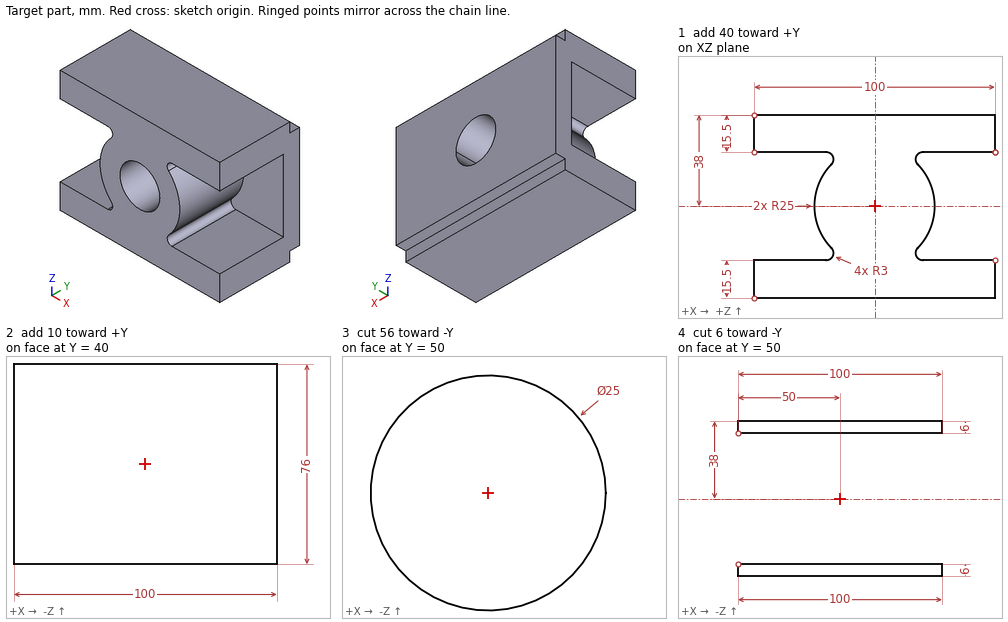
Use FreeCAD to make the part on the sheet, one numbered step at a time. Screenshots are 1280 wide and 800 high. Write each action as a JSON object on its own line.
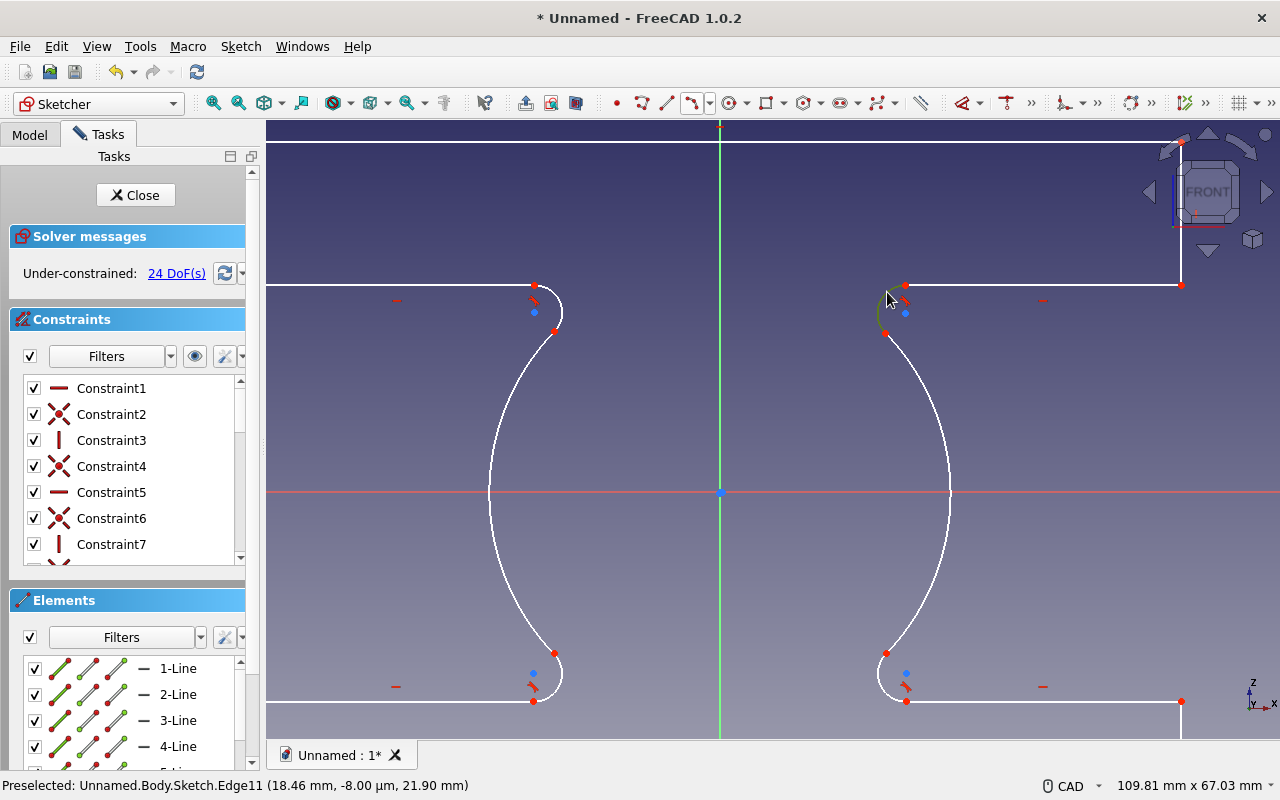
{"action": "left_click", "coordinate": [940, 563]}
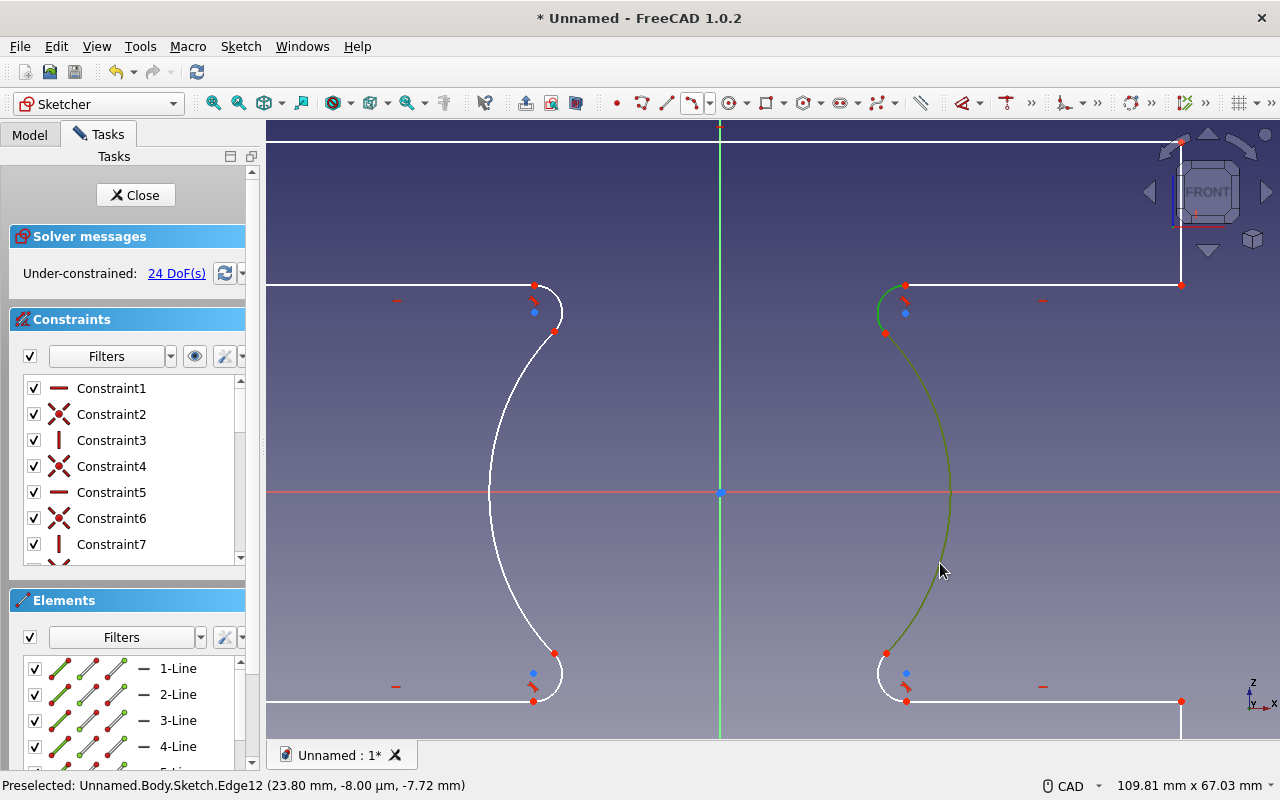
{"action": "key", "text": "t"}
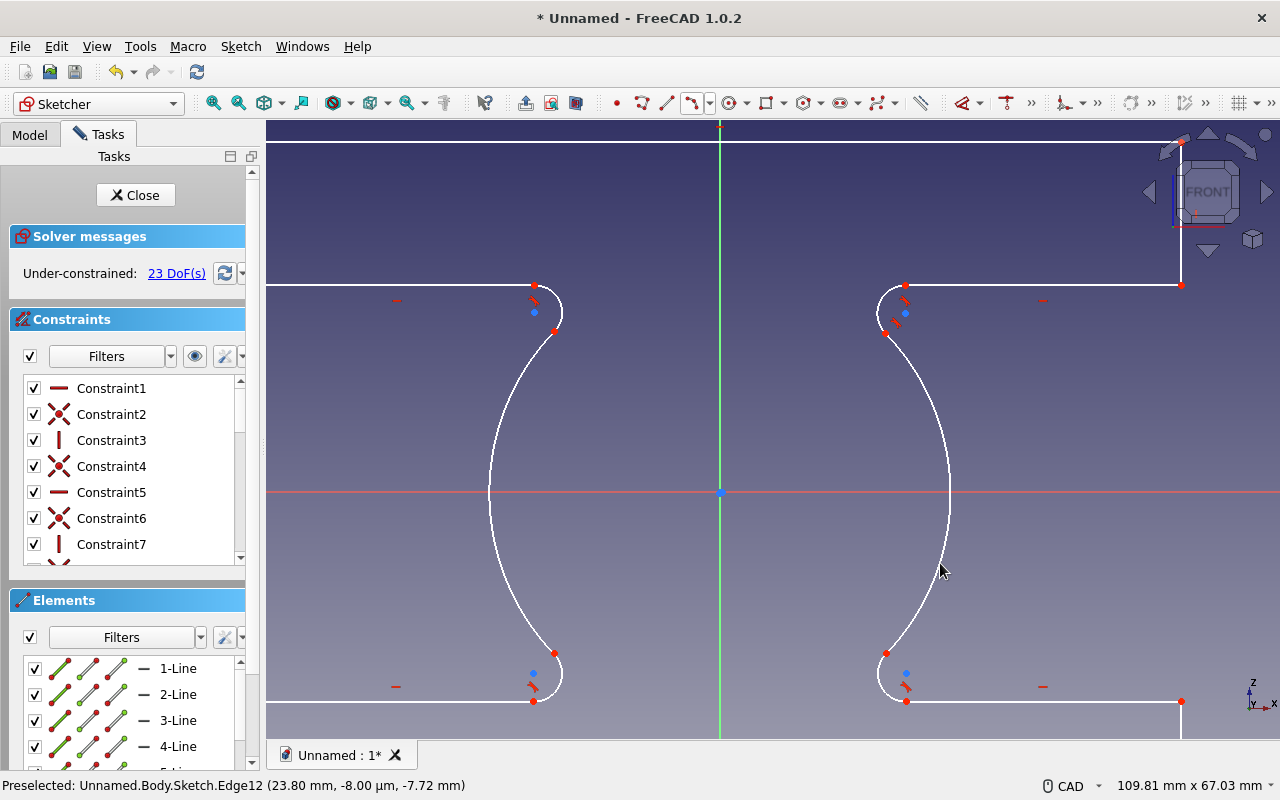
{"action": "left_click", "coordinate": [940, 563]}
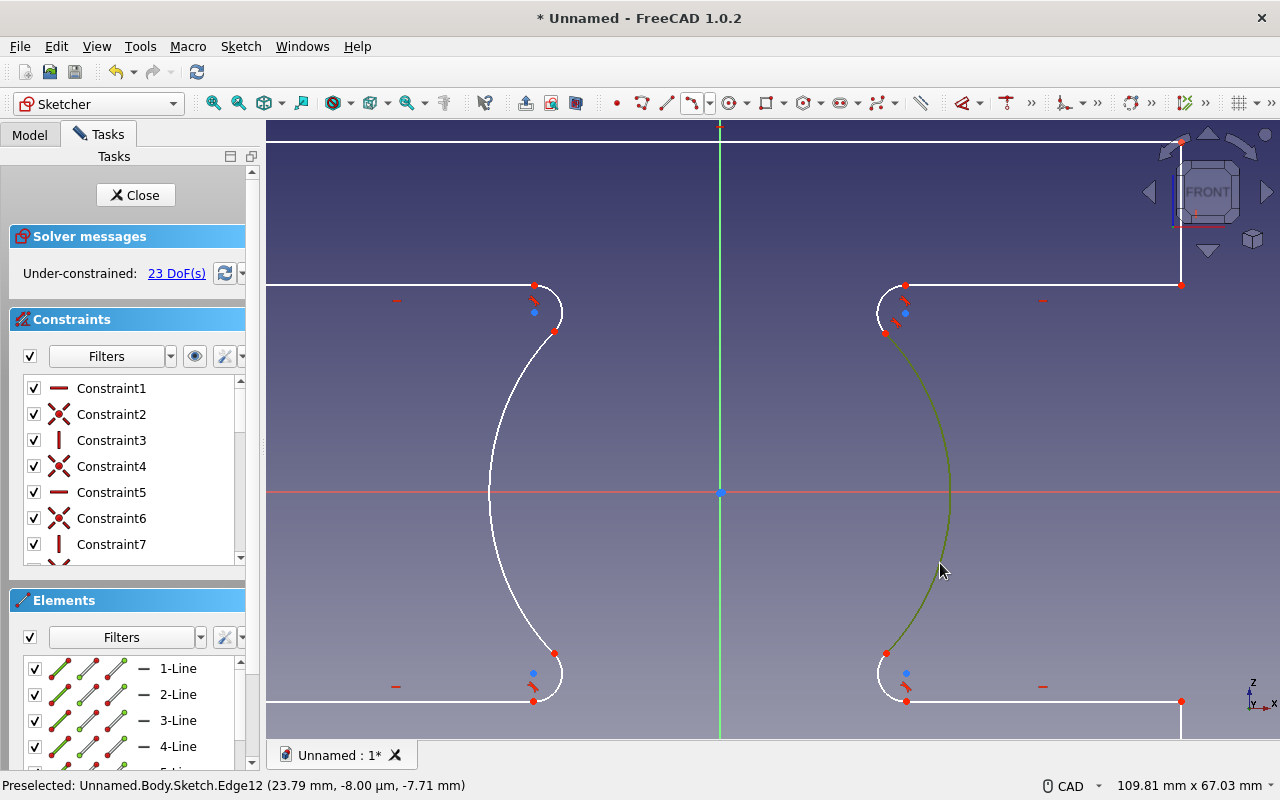
{"action": "left_click", "coordinate": [878, 672]}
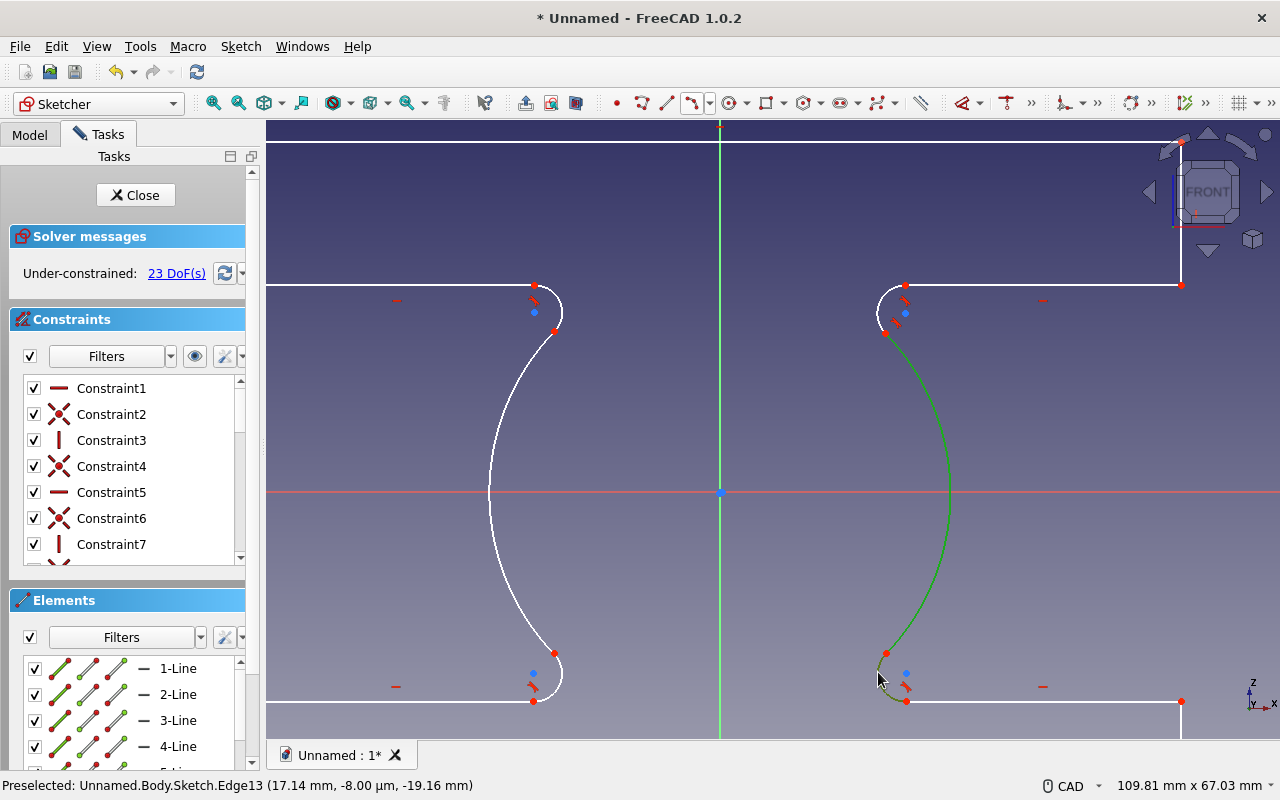
{"action": "key", "text": "t"}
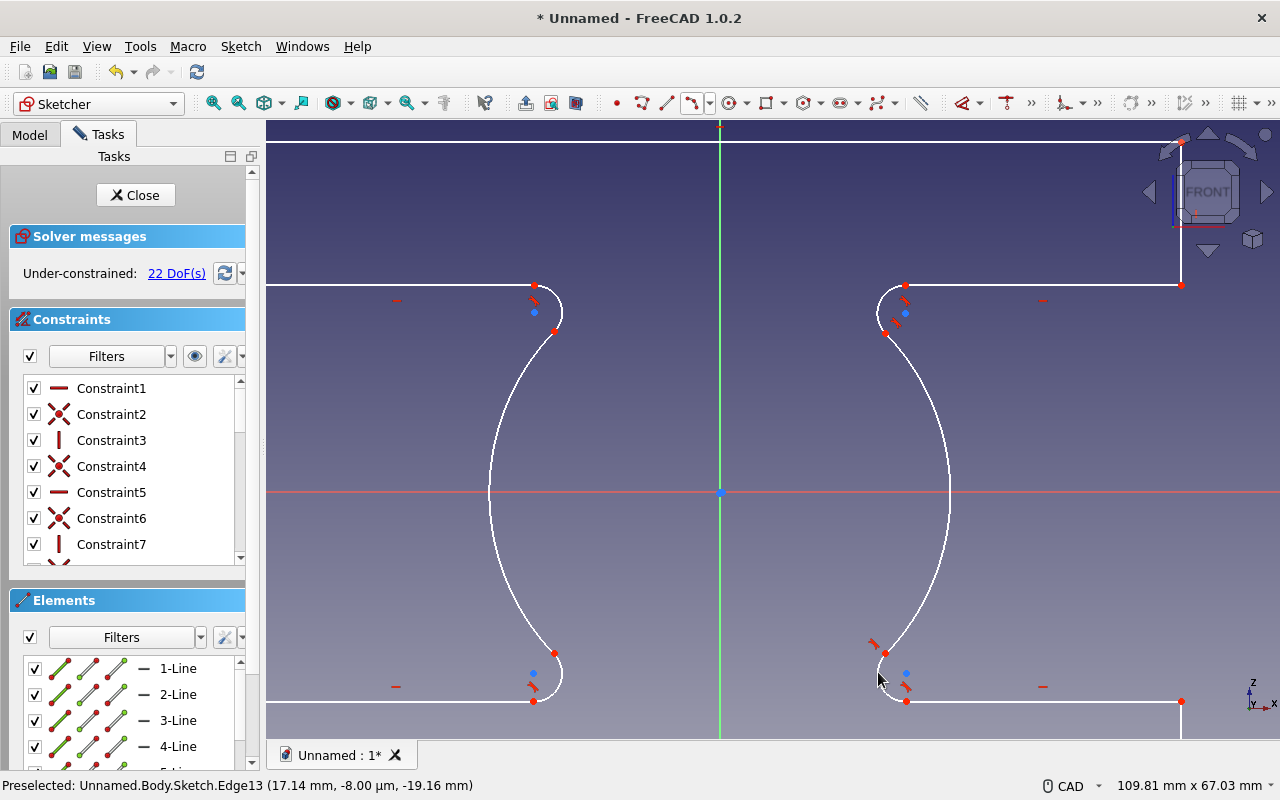
{"action": "left_click", "coordinate": [552, 695]}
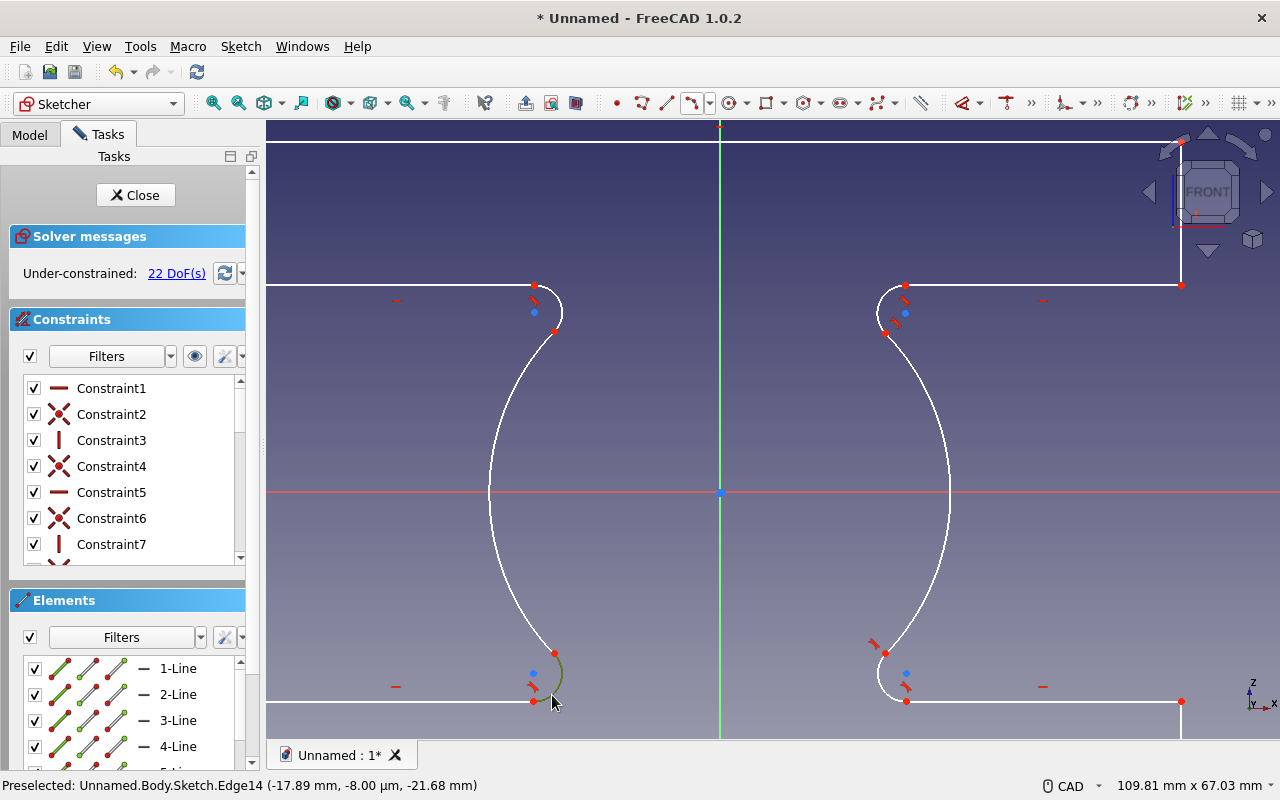
{"action": "left_click", "coordinate": [500, 423]}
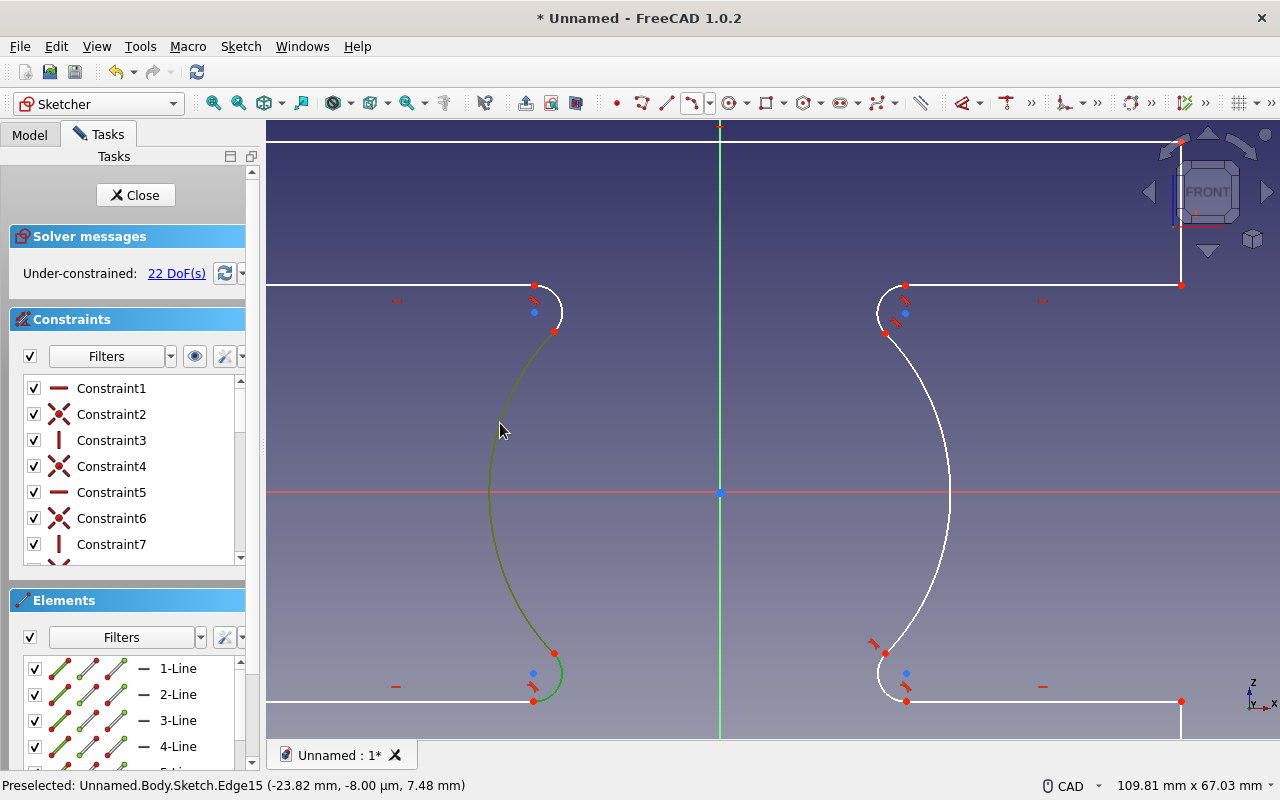
{"action": "key", "text": "t"}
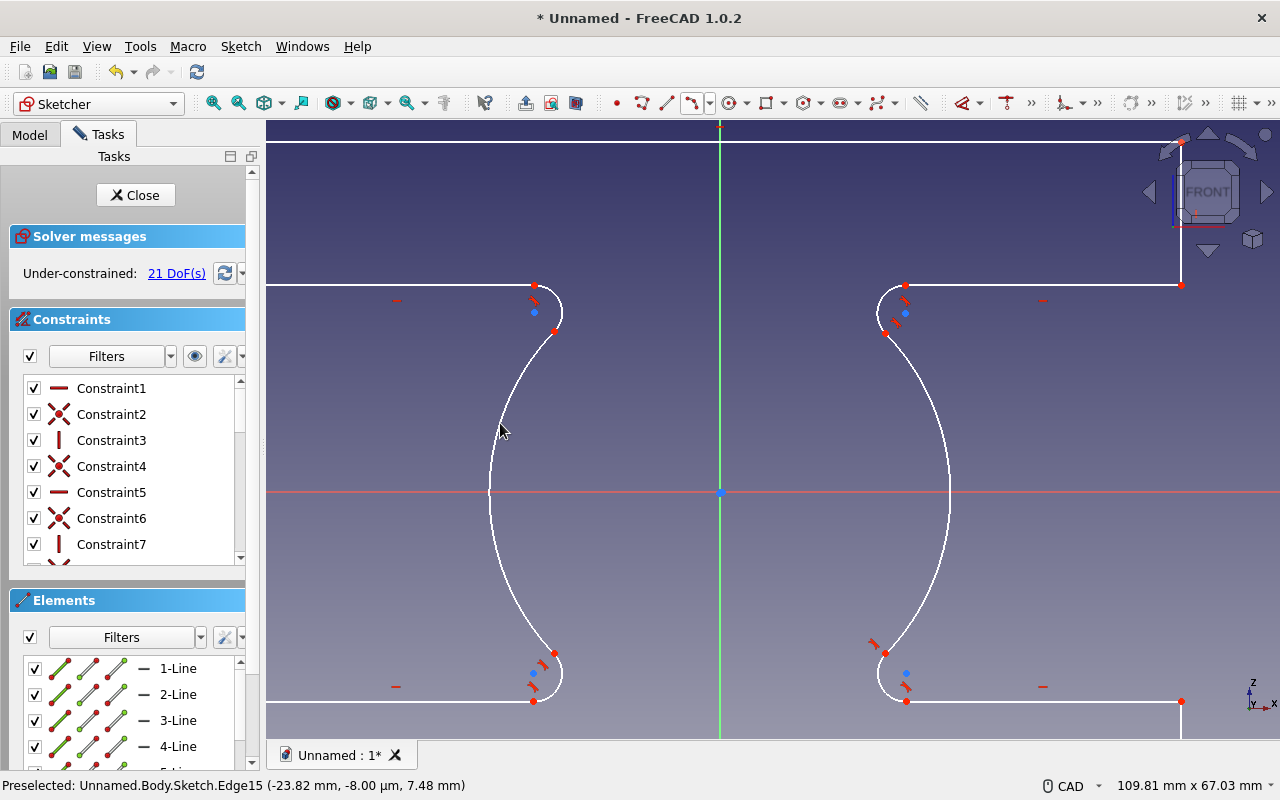
{"action": "left_click", "coordinate": [500, 423]}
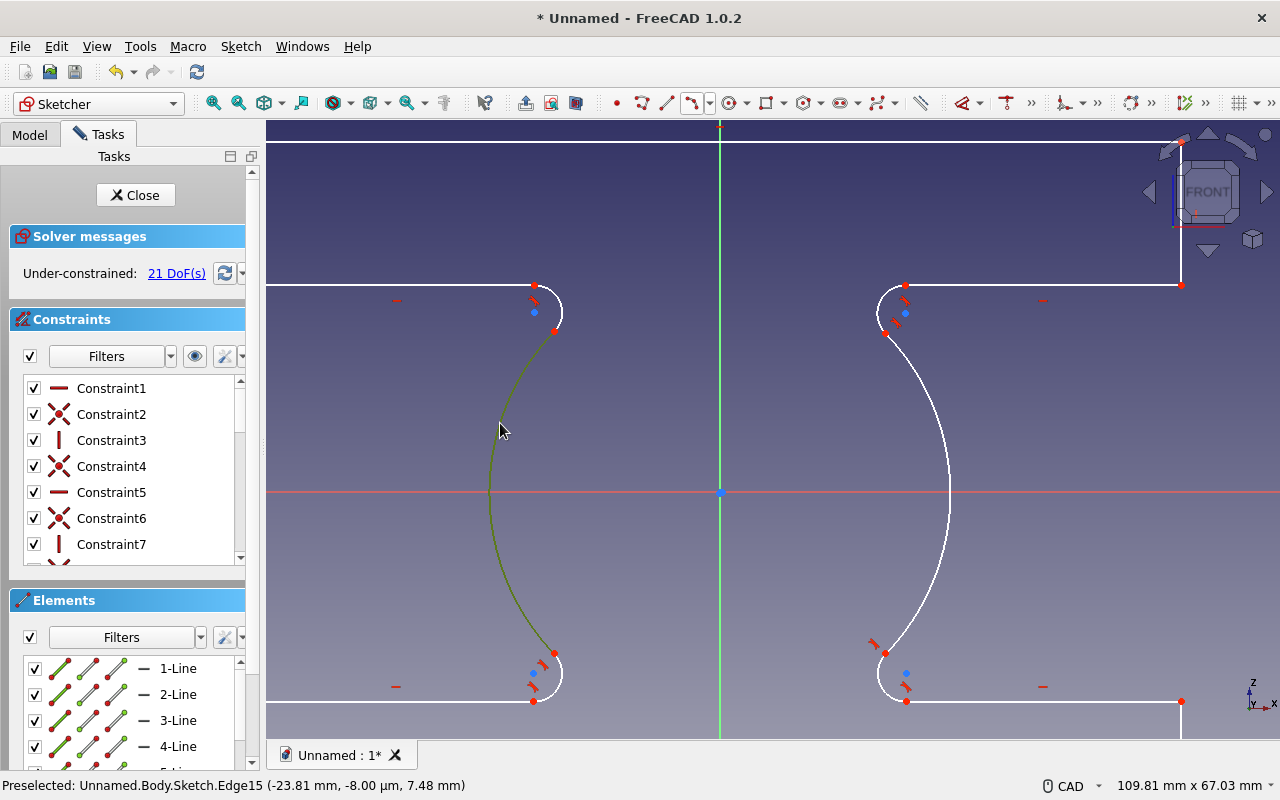
{"action": "left_click", "coordinate": [562, 315]}